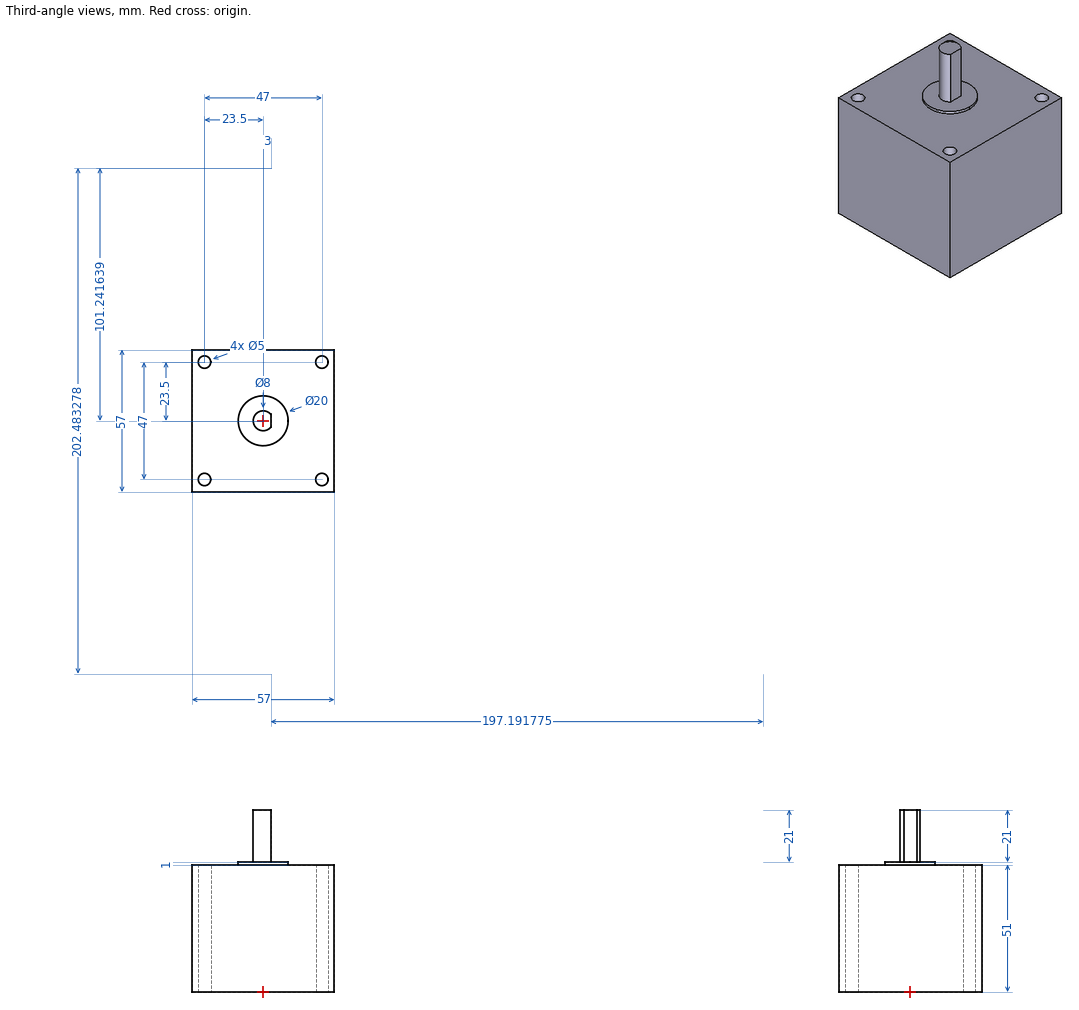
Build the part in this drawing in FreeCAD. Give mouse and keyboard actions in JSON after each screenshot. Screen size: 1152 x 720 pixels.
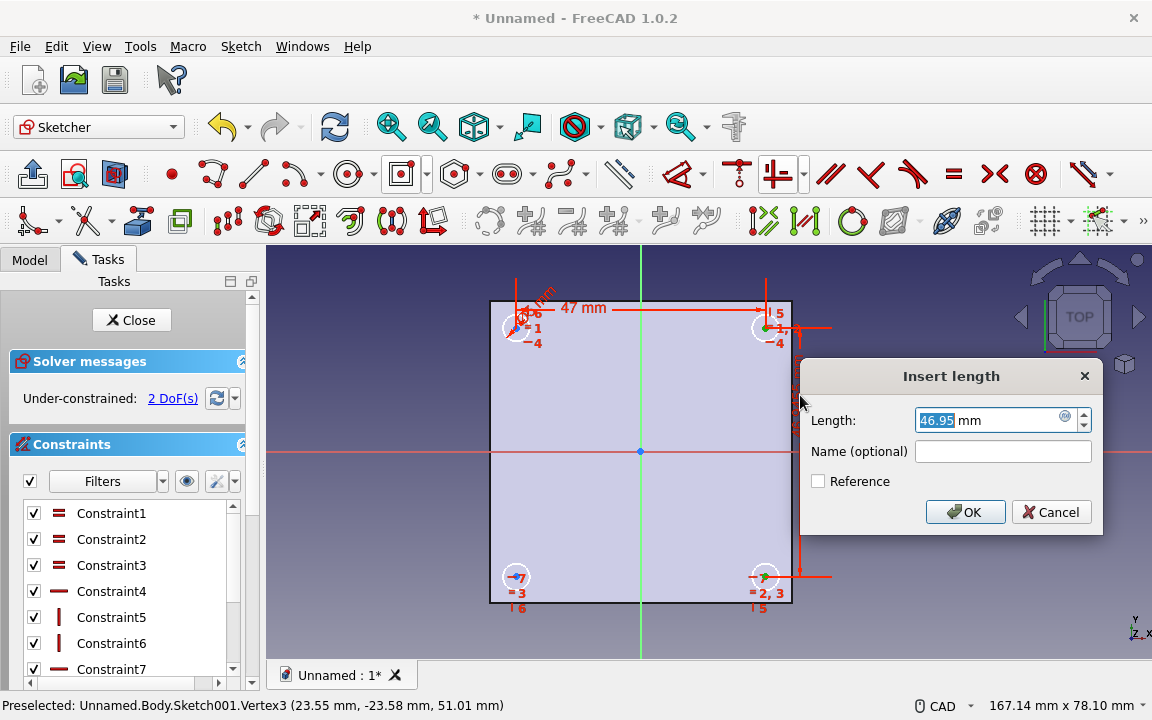
{"action": "type", "text": "47"}
{"action": "key", "text": "Return"}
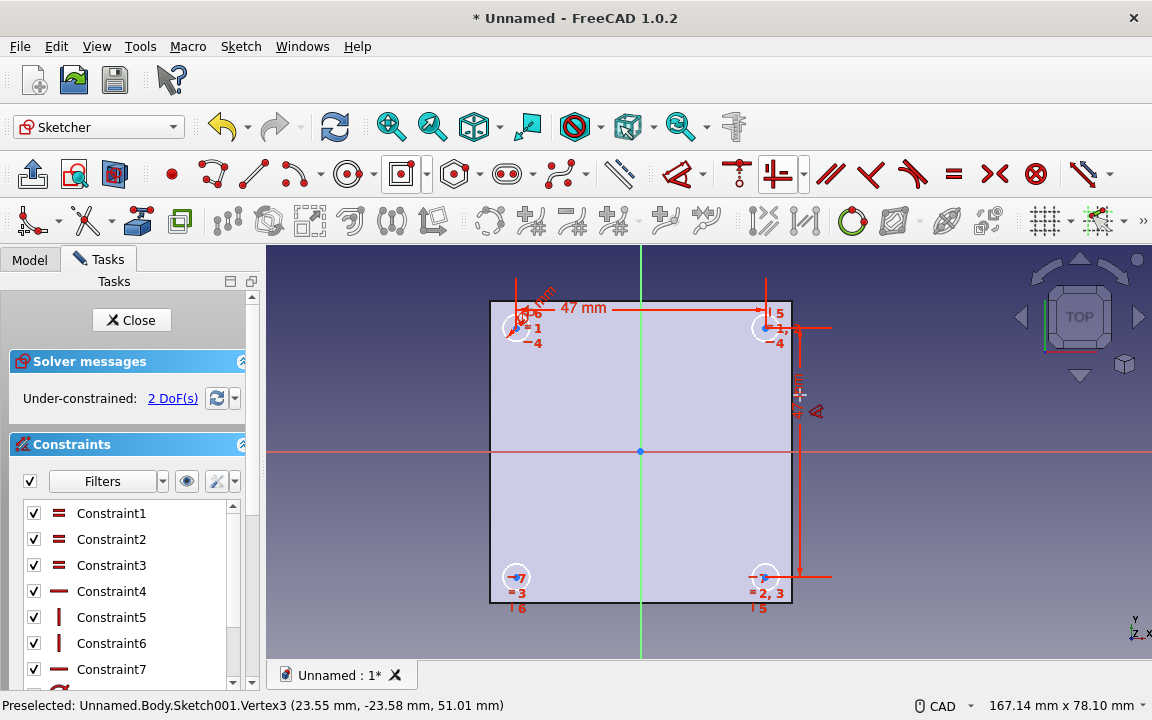
{"action": "left_click", "coordinate": [516, 328]}
{"action": "left_click", "coordinate": [579, 486]}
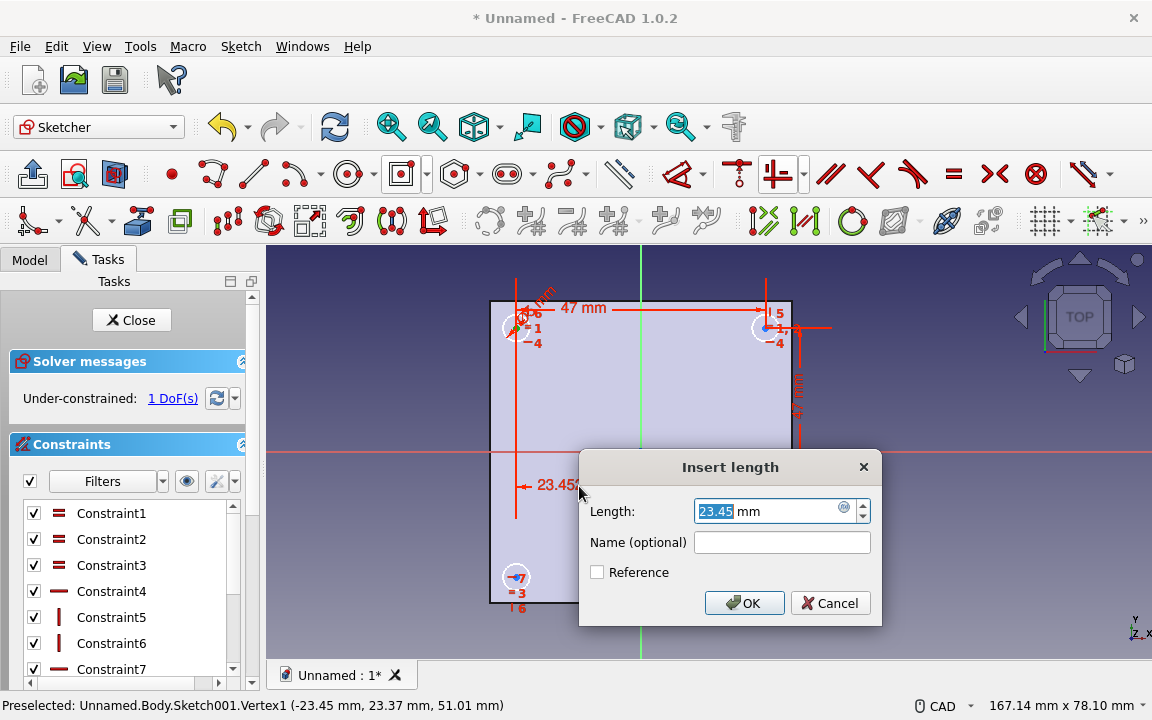
{"action": "type", "text": "23.5"}
{"action": "key", "text": "Return"}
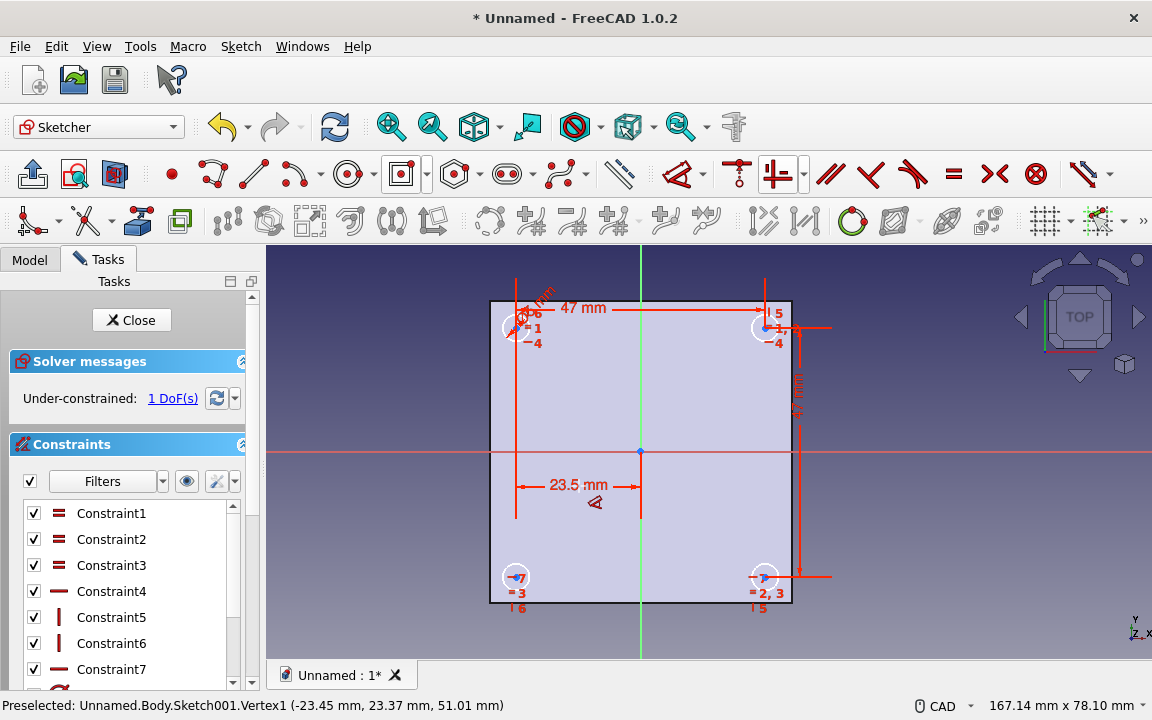
{"action": "left_click", "coordinate": [516, 328]}
{"action": "left_click", "coordinate": [482, 390]}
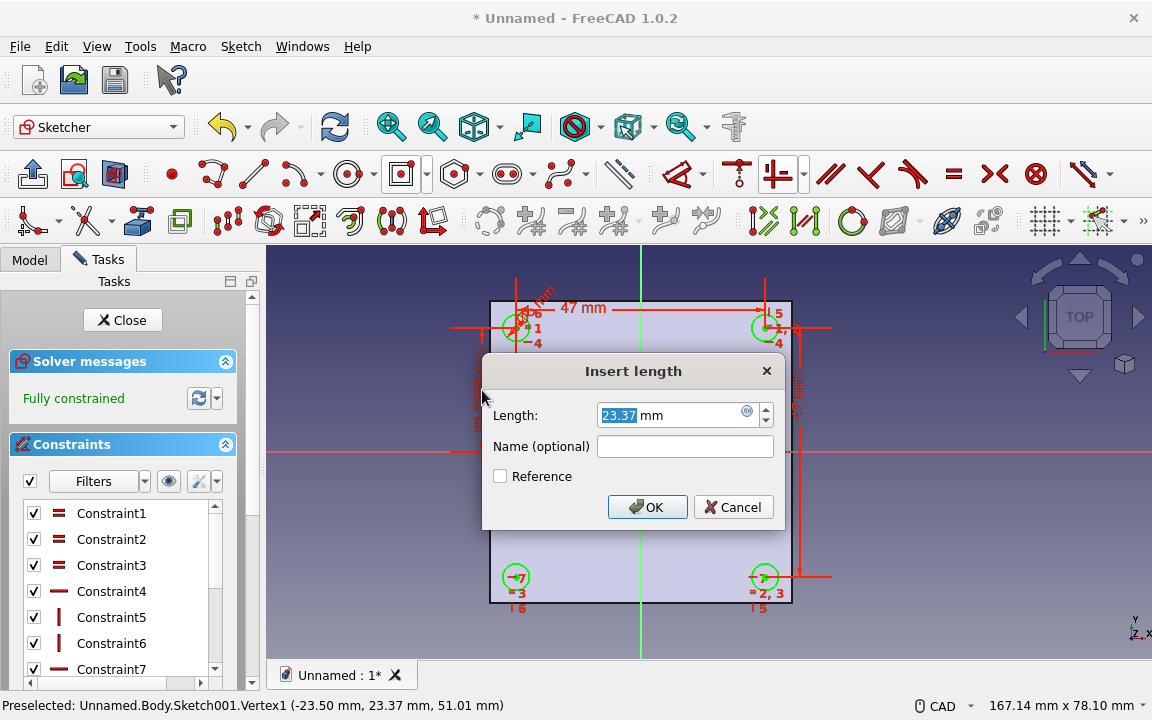
{"action": "type", "text": "23.5"}
{"action": "key", "text": "Return"}
{"action": "key", "text": "Escape"}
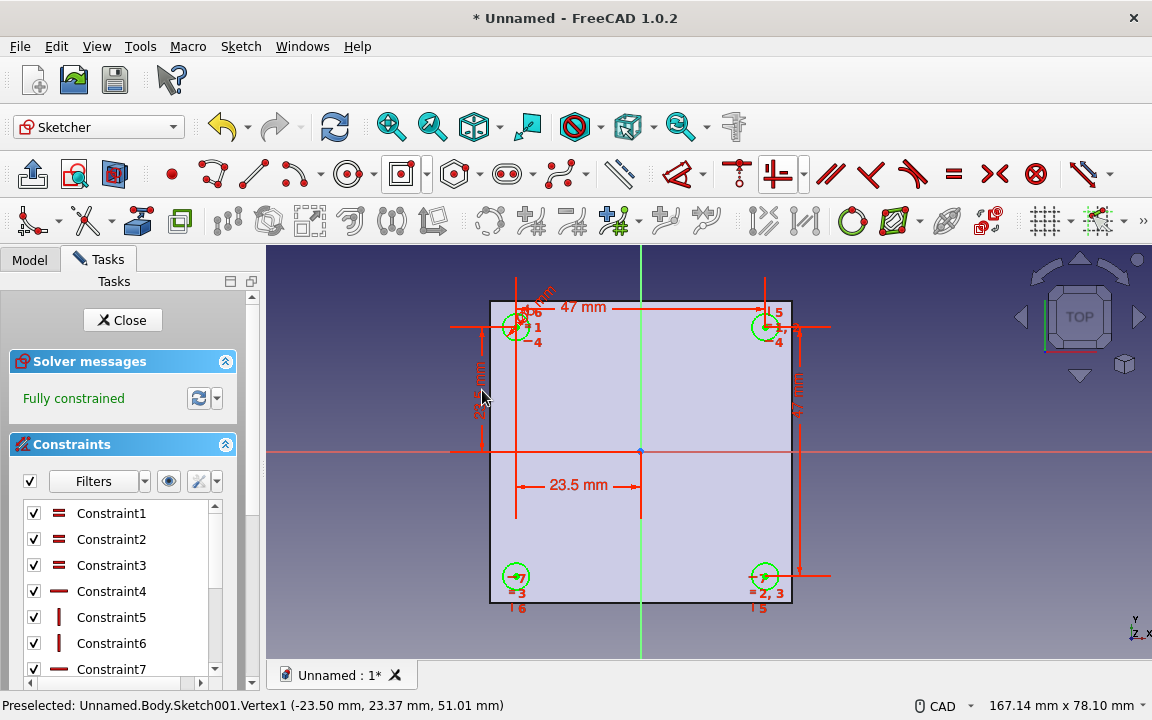
{"action": "left_click", "coordinate": [123, 320]}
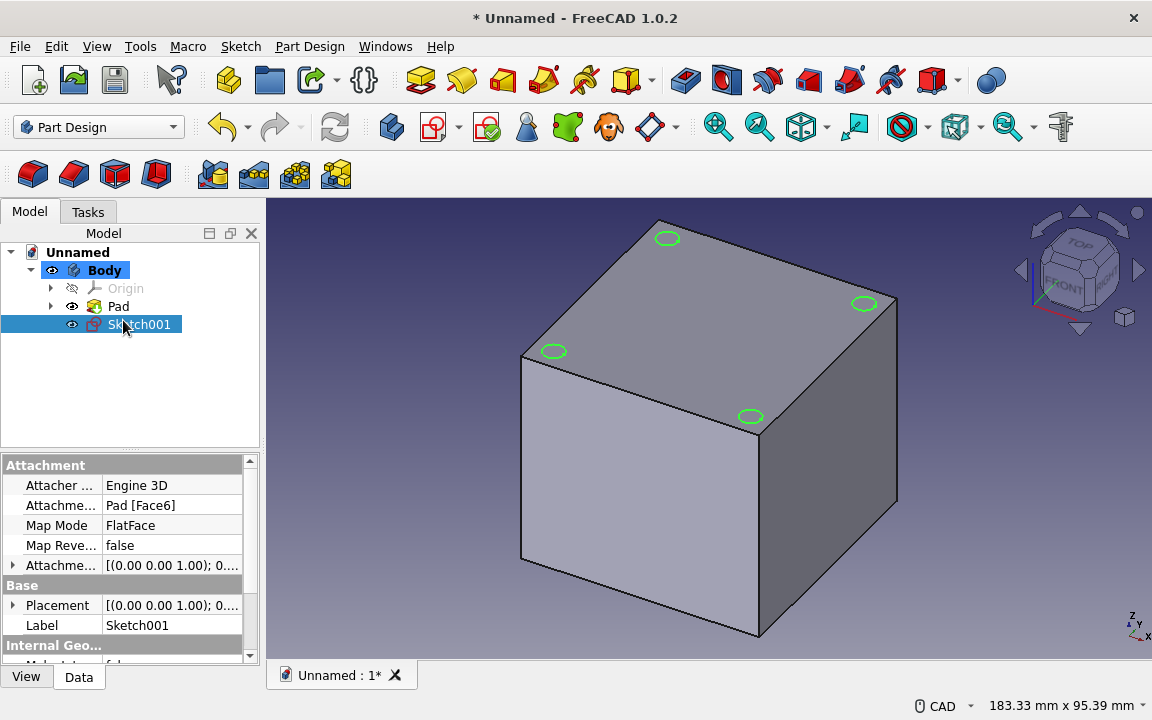
{"action": "left_click", "coordinate": [686, 80]}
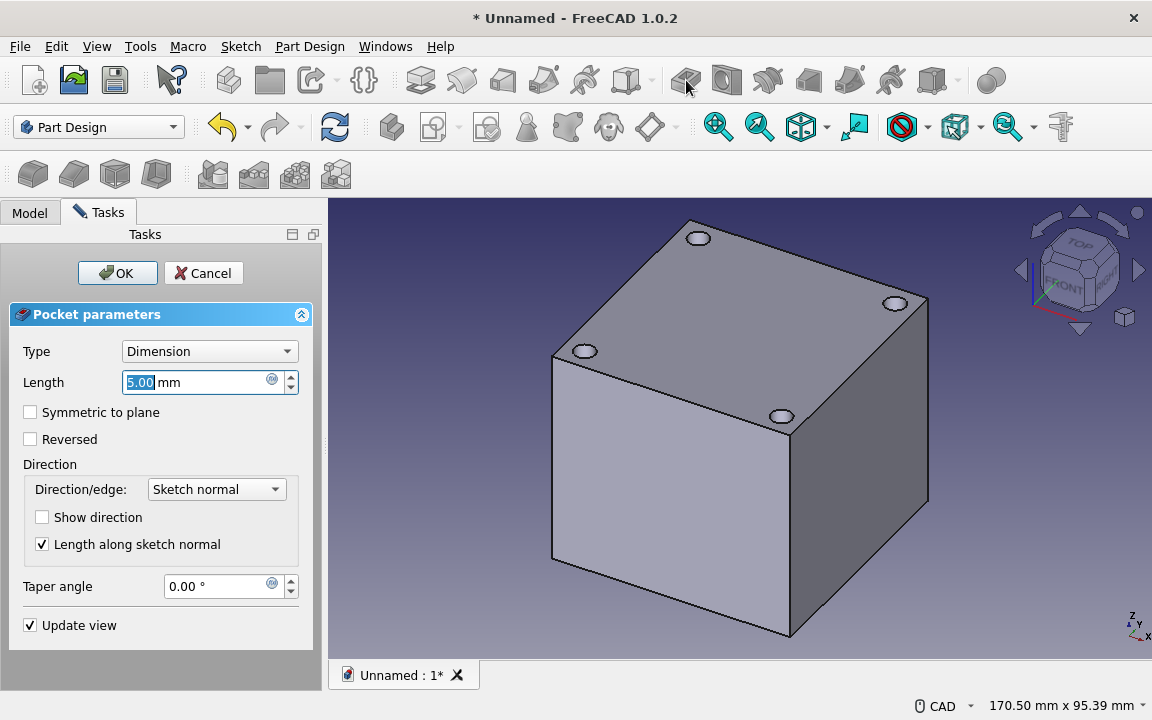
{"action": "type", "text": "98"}
{"action": "key", "text": "Tab"}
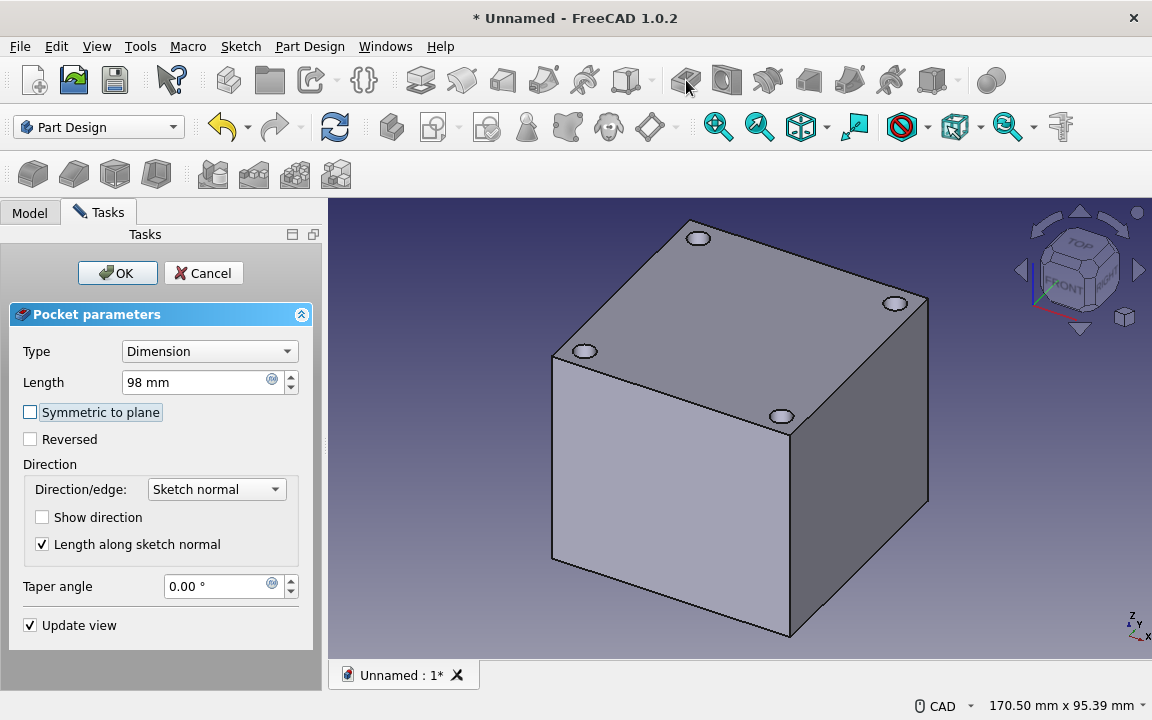
{"action": "left_click", "coordinate": [118, 273]}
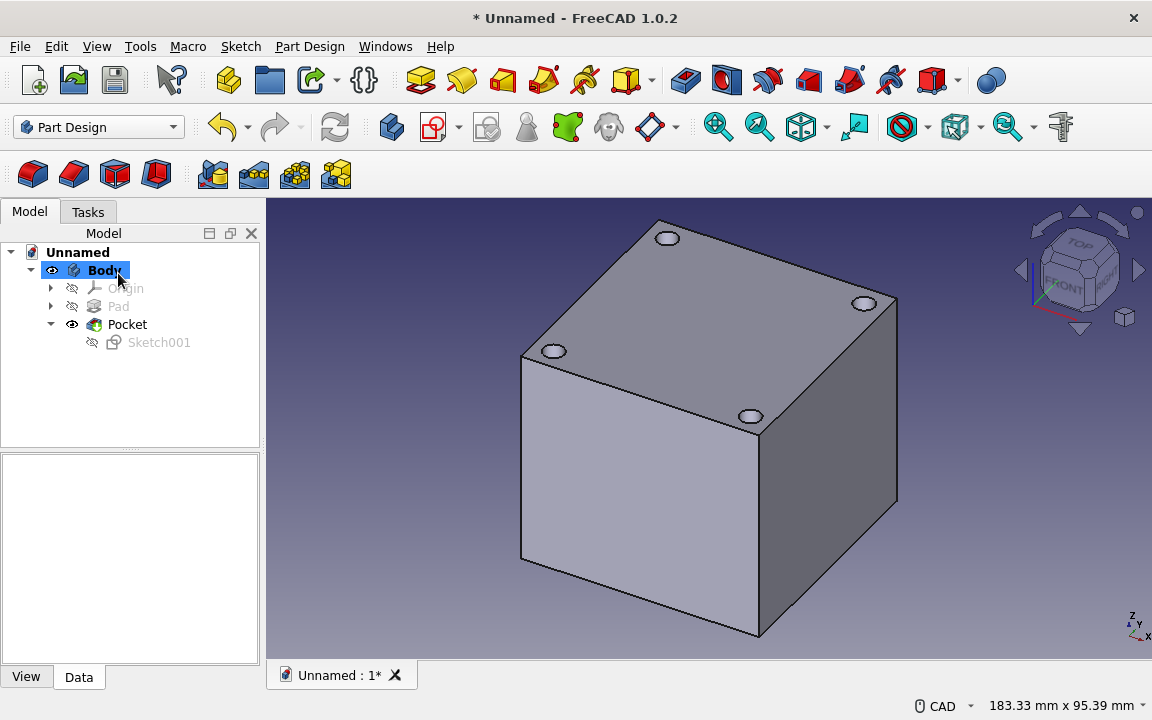
{"action": "left_click", "coordinate": [709, 327]}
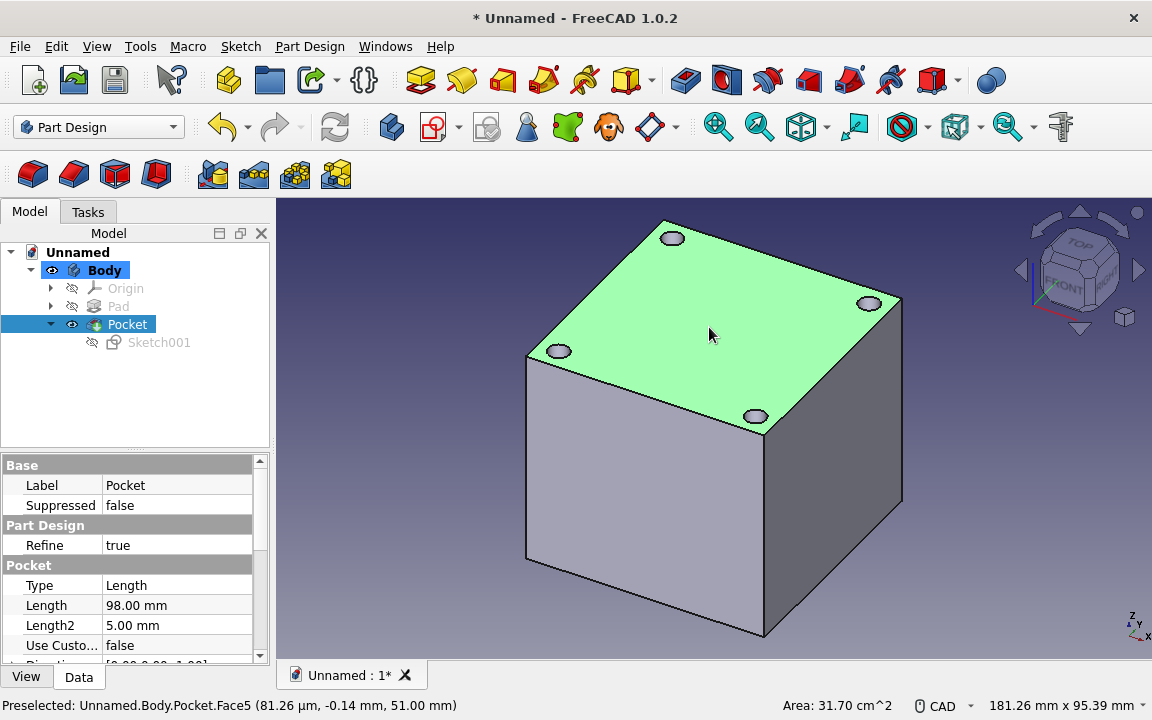
{"action": "left_click", "coordinate": [432, 128]}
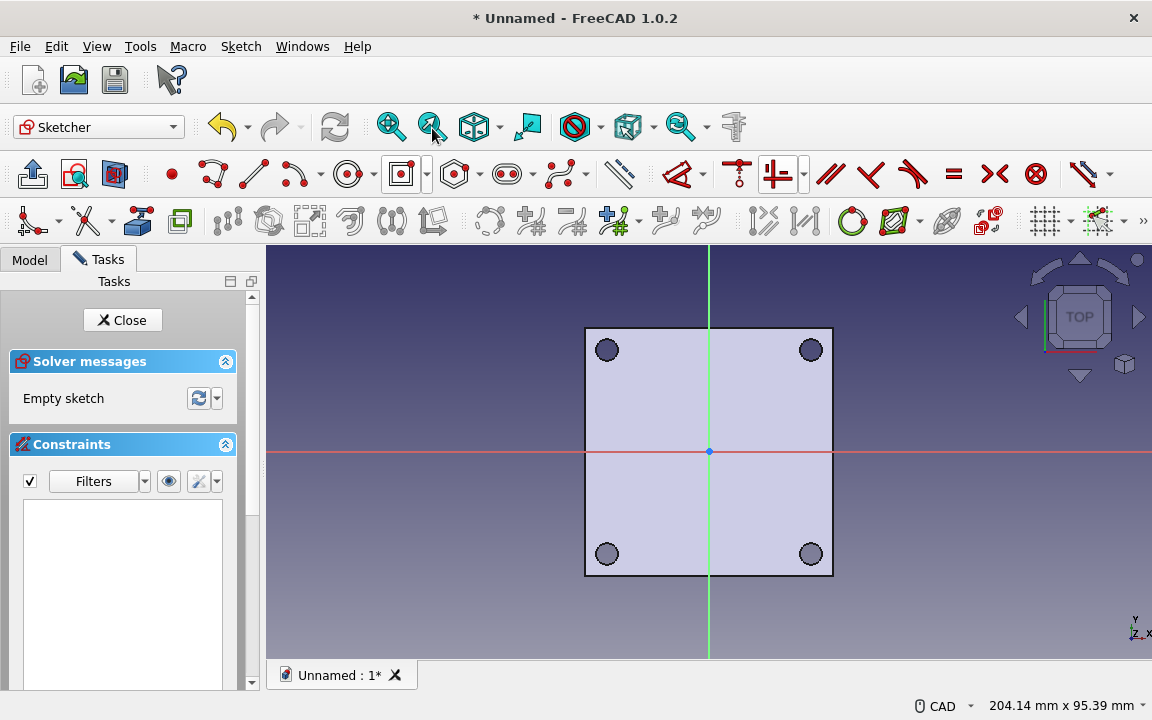
{"action": "scroll", "coordinate": [749, 452], "scroll_direction": "up", "scroll_amount": 5}